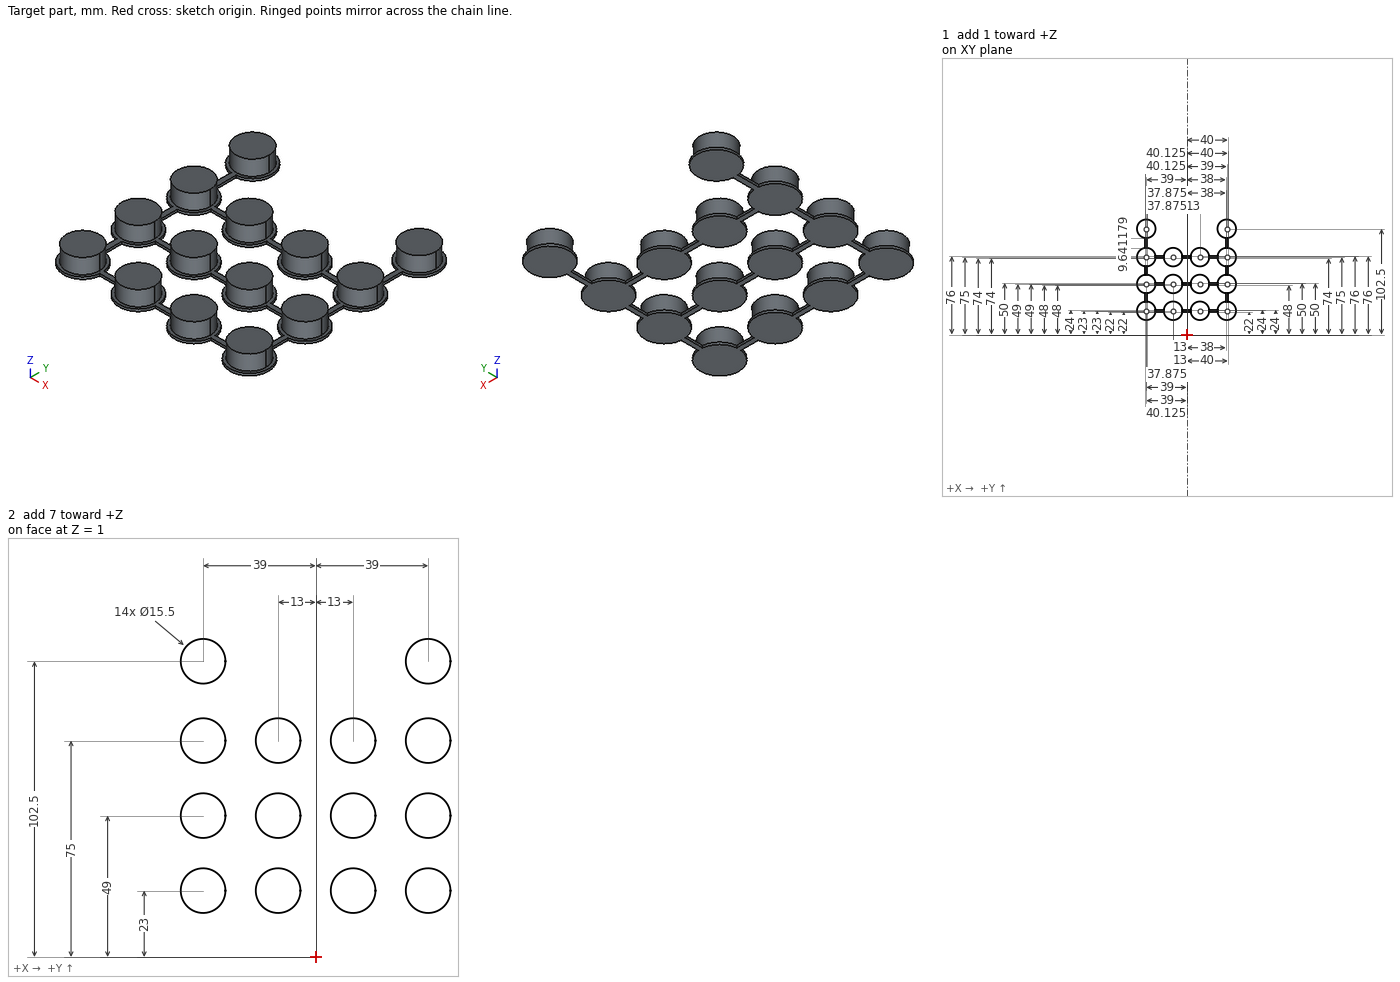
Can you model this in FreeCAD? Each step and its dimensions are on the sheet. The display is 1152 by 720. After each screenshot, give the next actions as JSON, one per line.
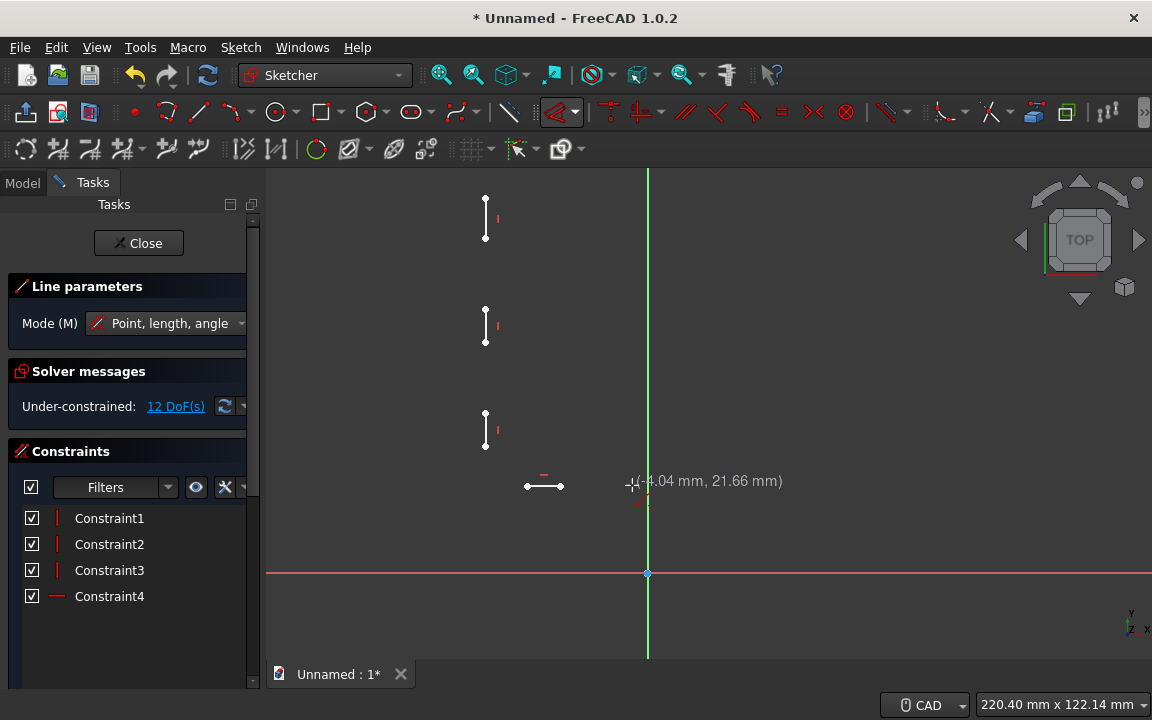
{"action": "left_click", "coordinate": [632, 485]}
{"action": "left_click", "coordinate": [664, 485]}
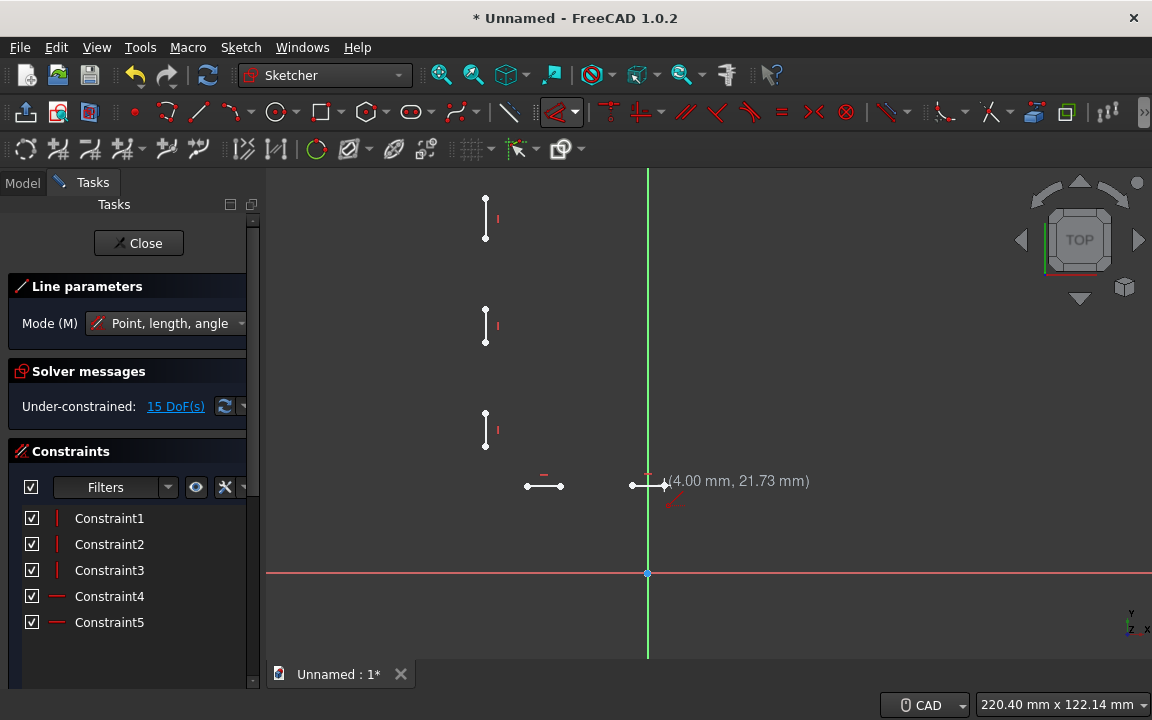
{"action": "left_click", "coordinate": [736, 485]}
{"action": "left_click", "coordinate": [769, 485]}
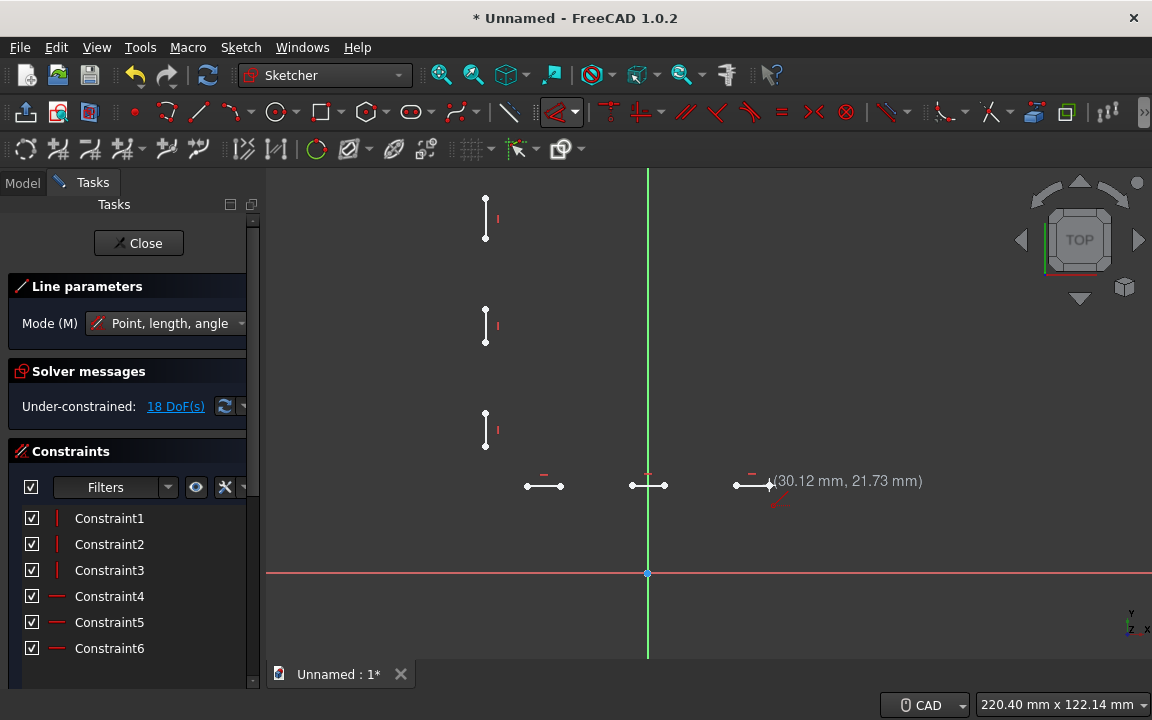
{"action": "left_click", "coordinate": [809, 445]}
{"action": "left_click", "coordinate": [809, 412]}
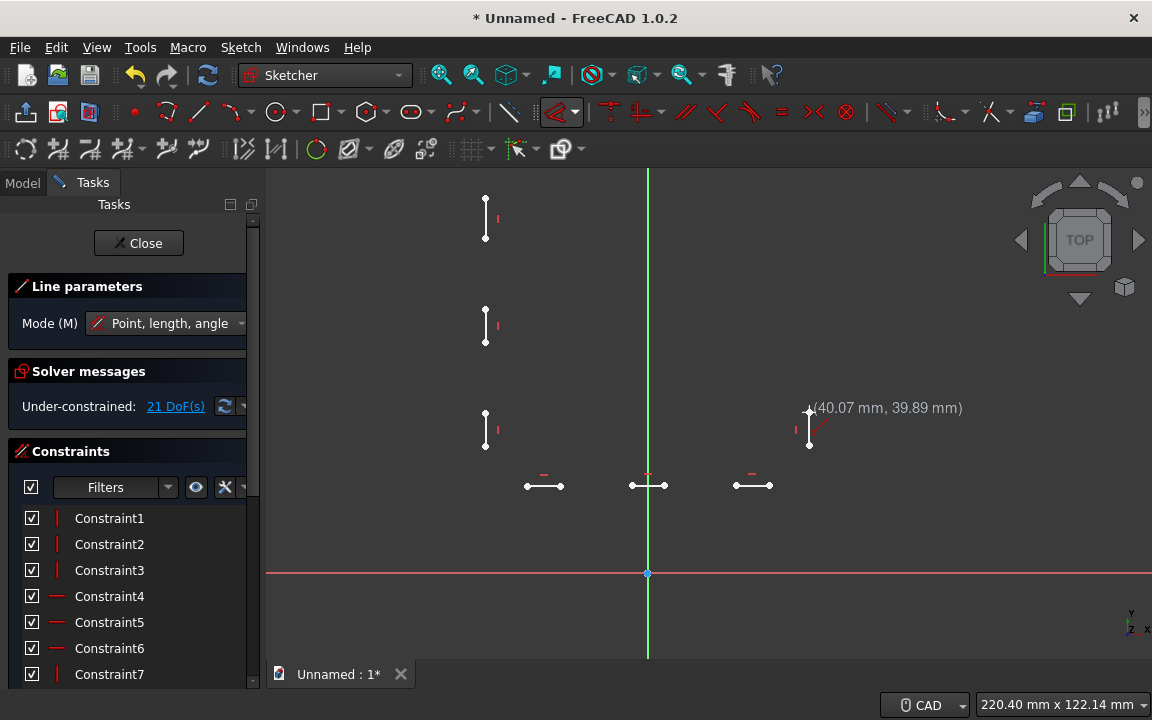
{"action": "left_click", "coordinate": [809, 340]}
{"action": "left_click", "coordinate": [809, 308]}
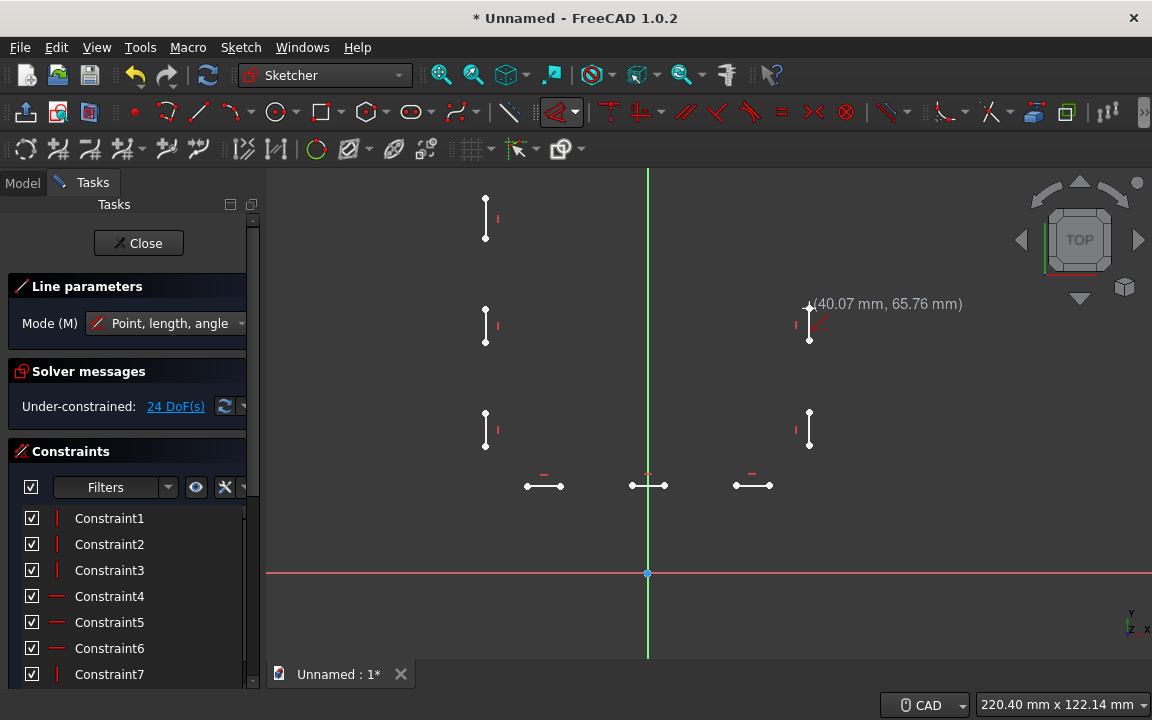
{"action": "left_click", "coordinate": [809, 236]}
{"action": "left_click", "coordinate": [809, 197]}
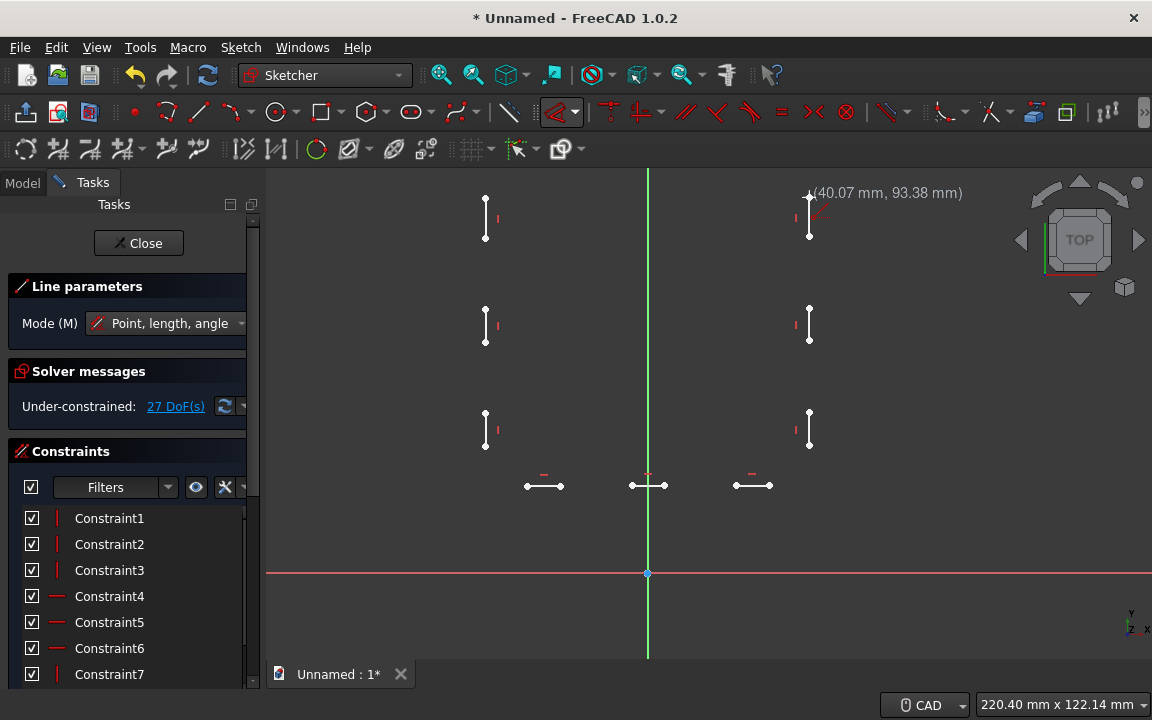
{"action": "scroll", "coordinate": [801, 197], "scroll_direction": "up", "scroll_amount": 4}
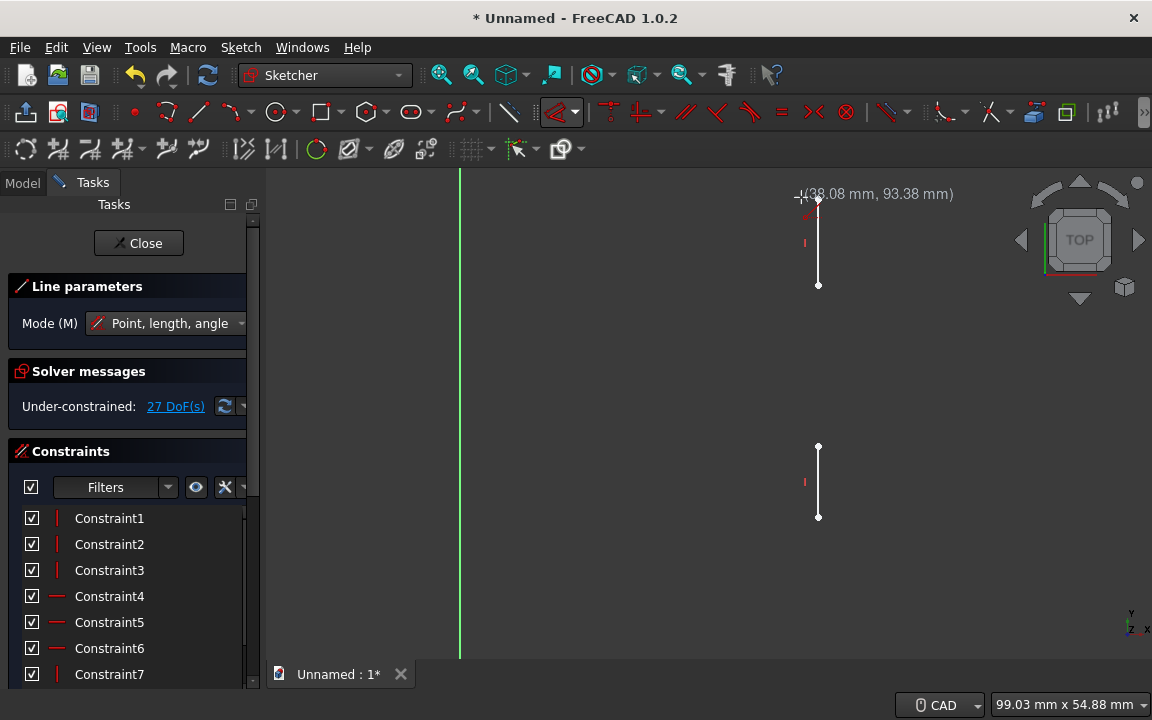
{"action": "left_click", "coordinate": [800, 198]}
{"action": "left_click", "coordinate": [800, 284]}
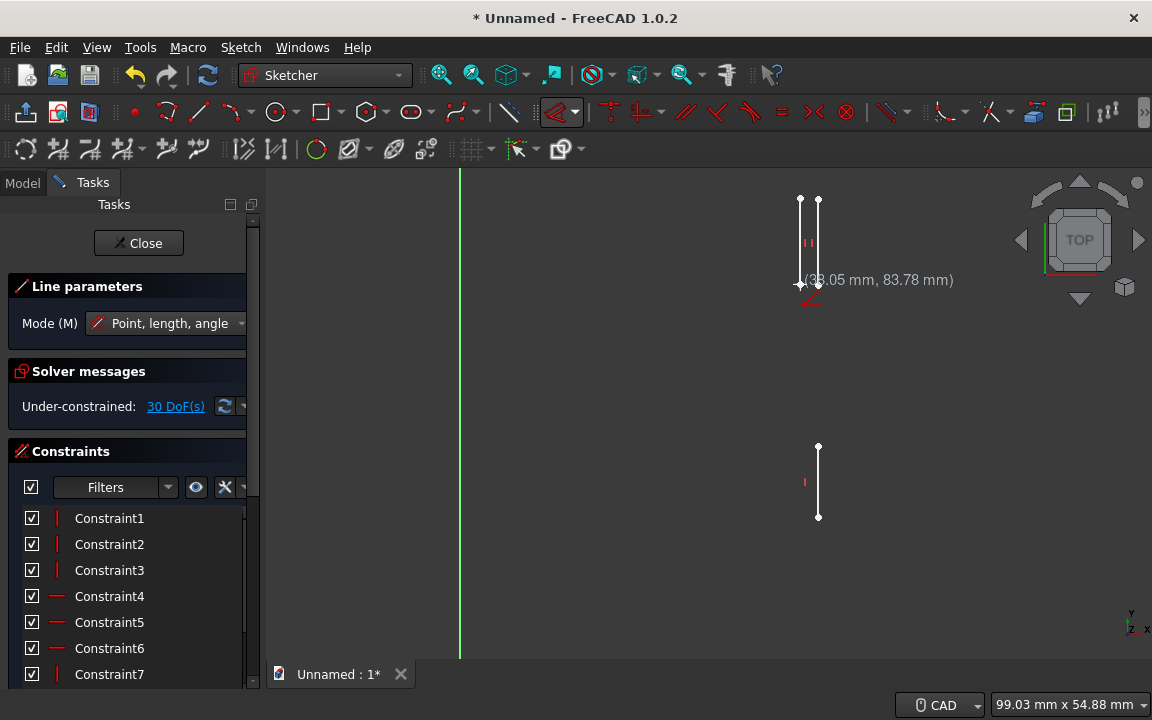
{"action": "scroll", "coordinate": [718, 361], "scroll_direction": "down", "scroll_amount": 6}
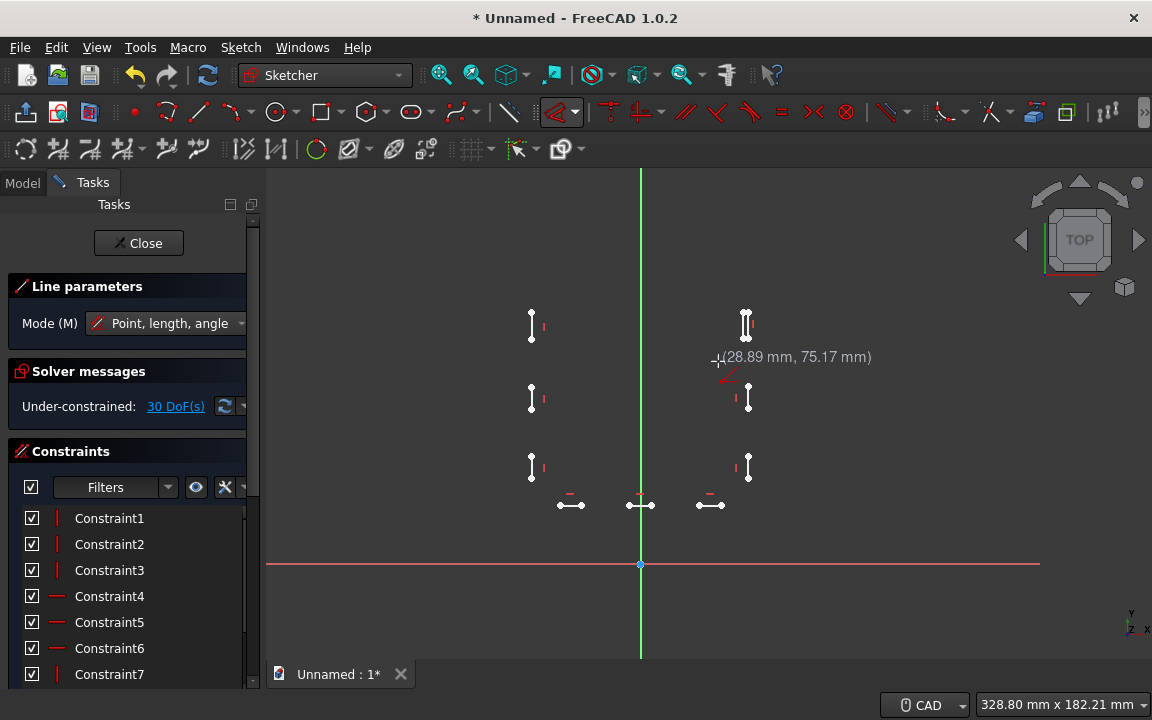
{"action": "left_click", "coordinate": [722, 359]}
{"action": "left_click", "coordinate": [700, 359]}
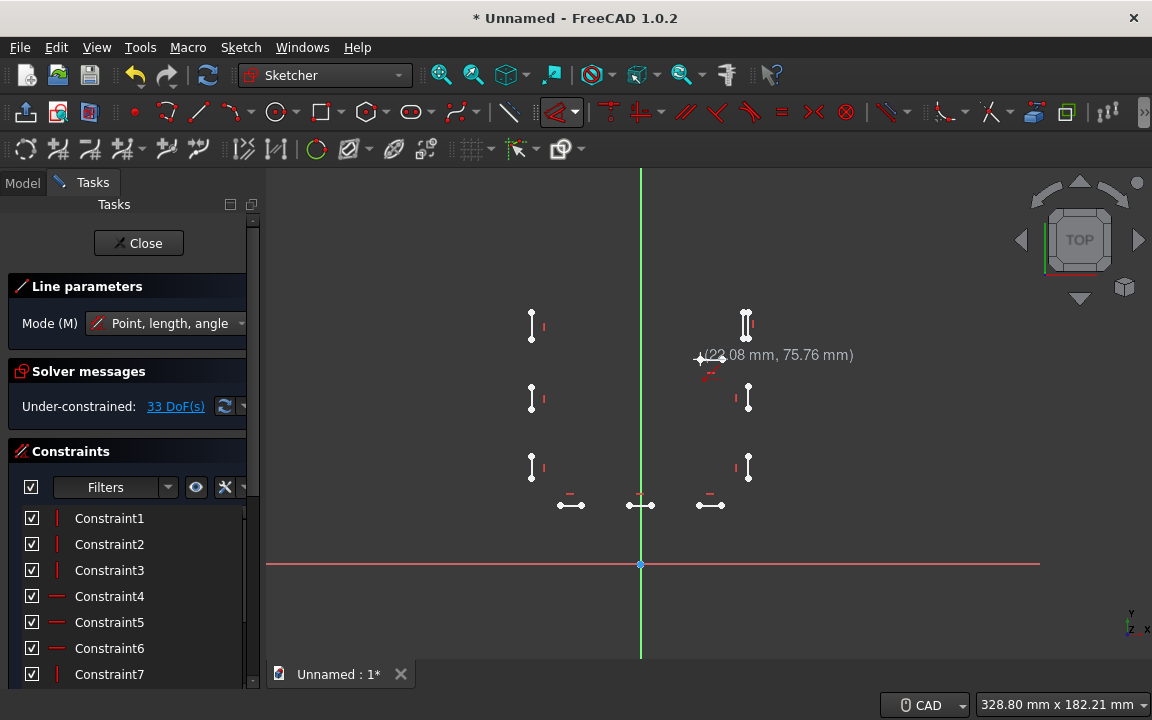
{"action": "scroll", "coordinate": [651, 359], "scroll_direction": "up", "scroll_amount": 2}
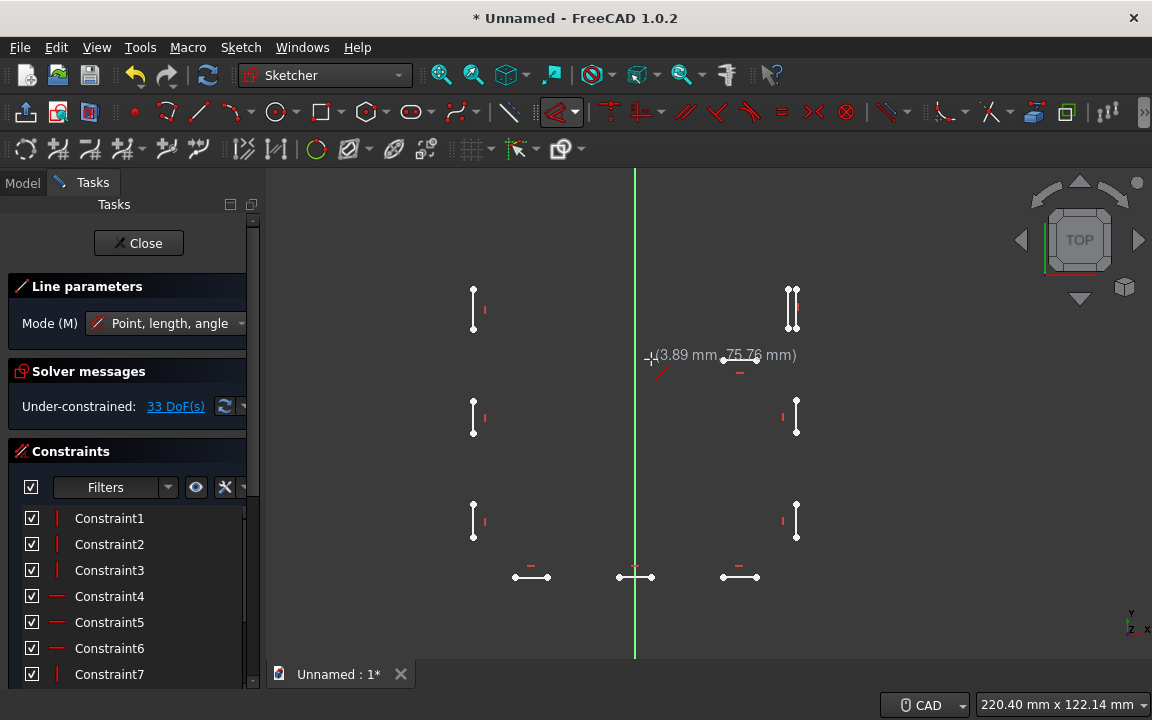
{"action": "left_click", "coordinate": [651, 359]}
{"action": "left_click", "coordinate": [619, 359]}